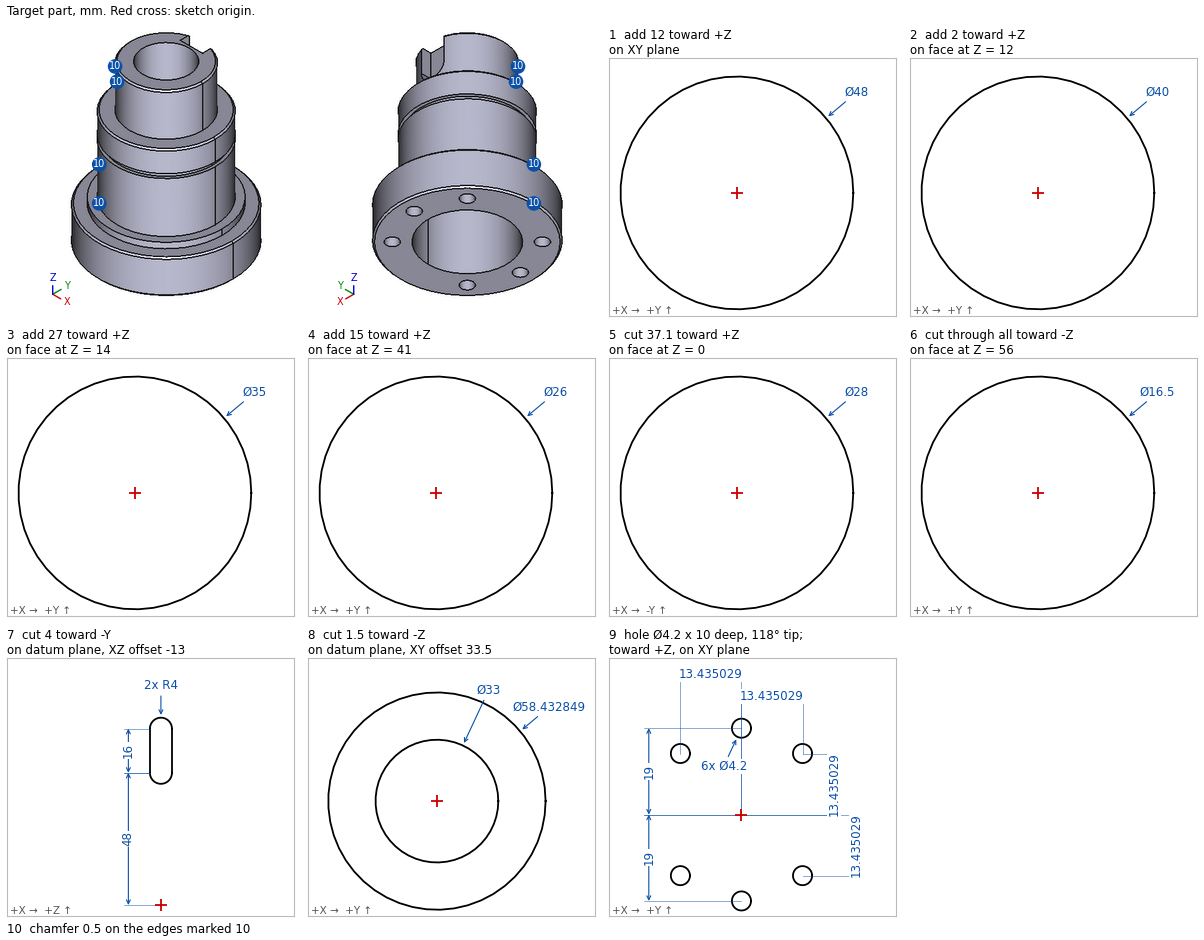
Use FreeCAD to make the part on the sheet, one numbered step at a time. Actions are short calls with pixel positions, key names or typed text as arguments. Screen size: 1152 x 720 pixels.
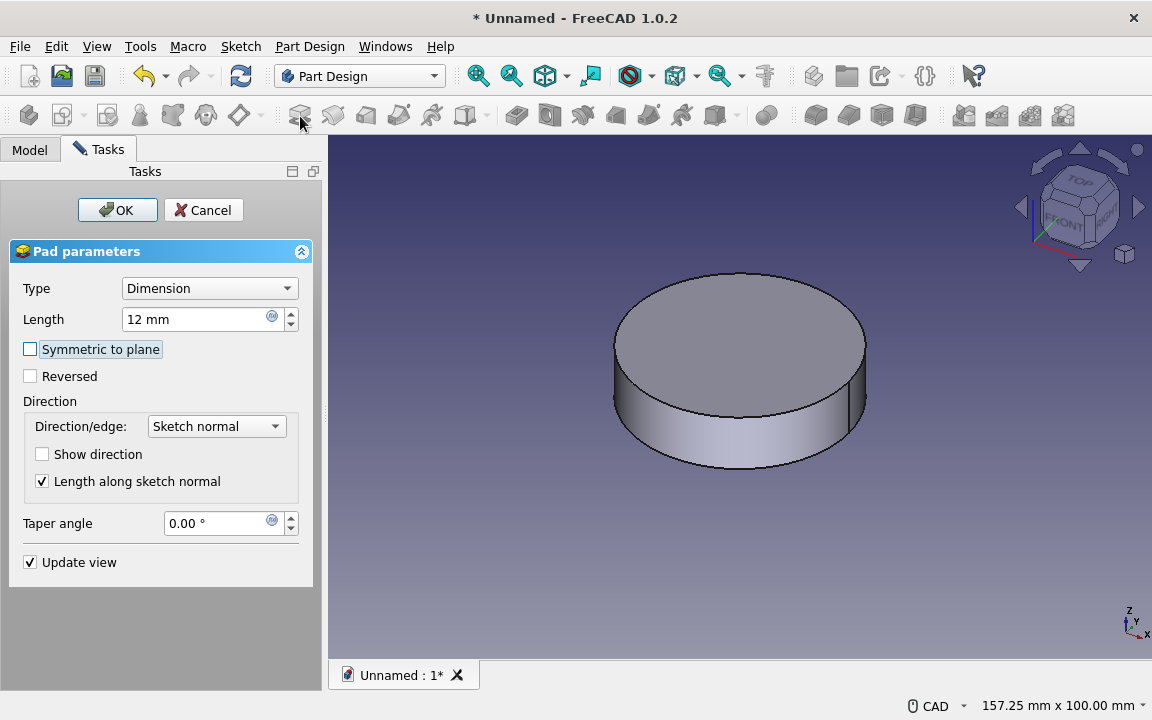
click(118, 210)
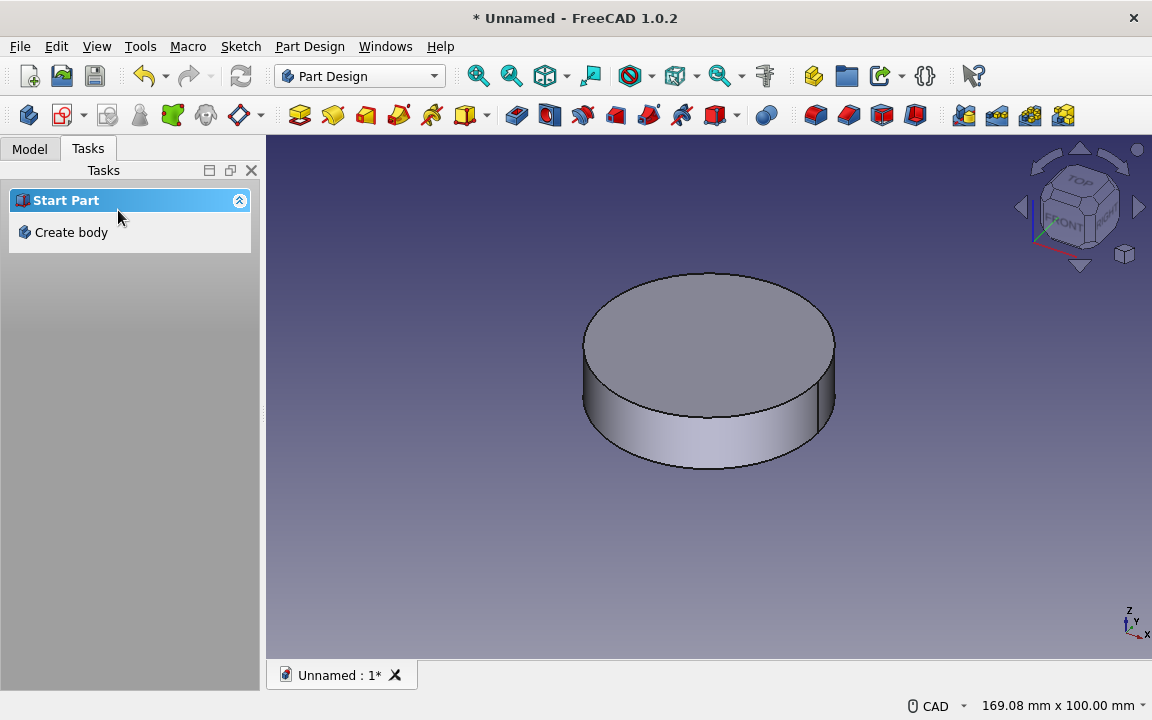
click(709, 344)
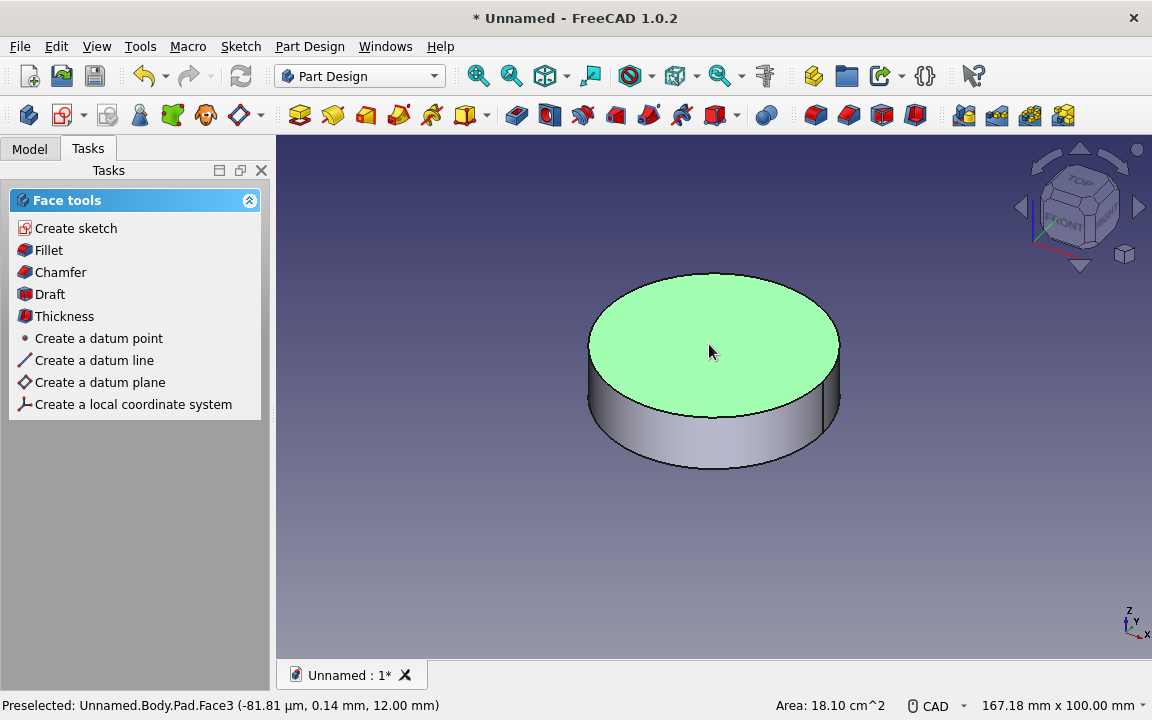
click(62, 116)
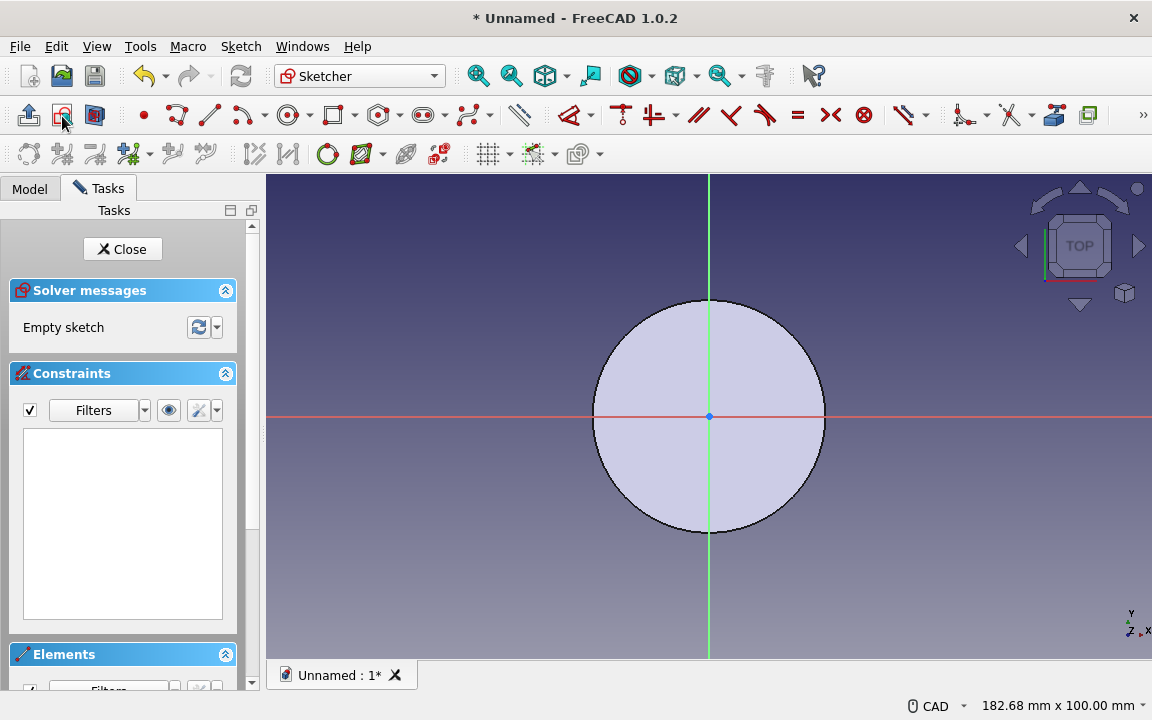
scroll(848, 416, up, 2)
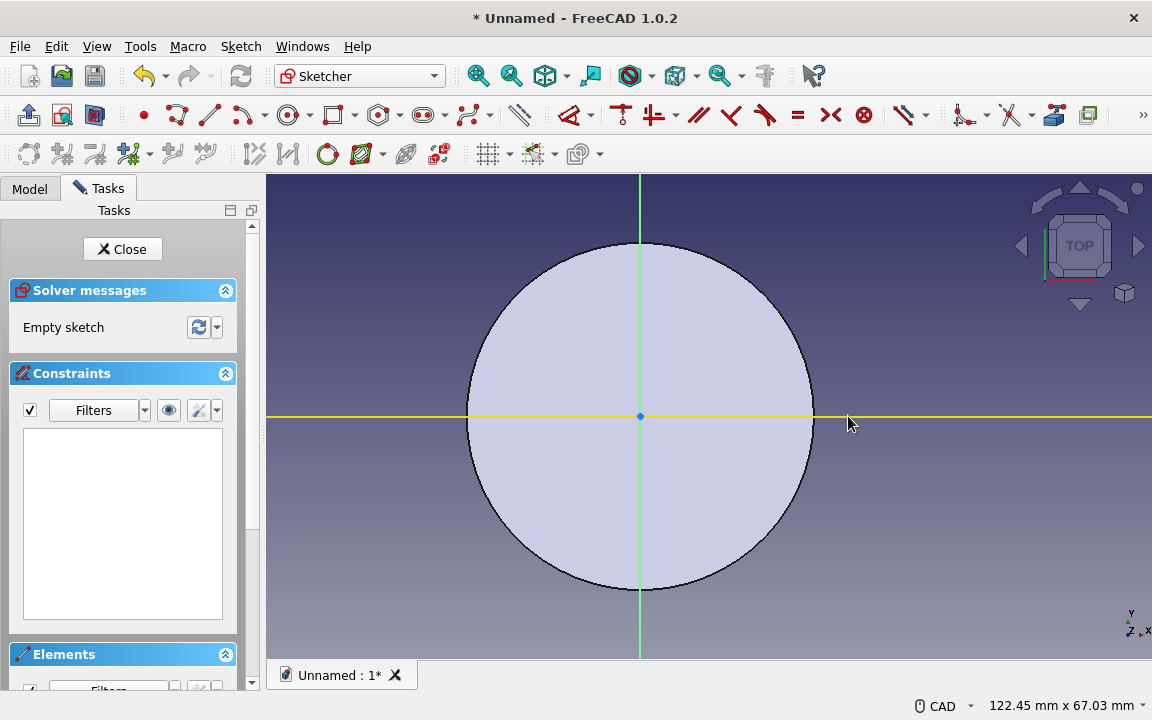
click(288, 116)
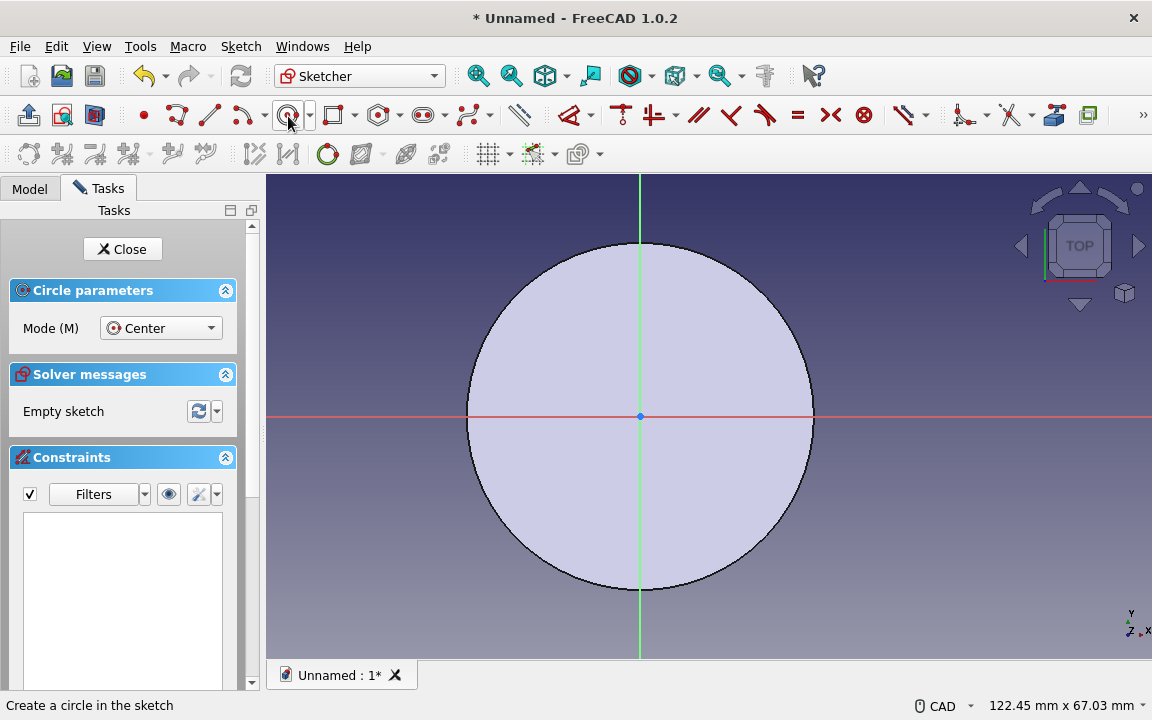
click(640, 416)
click(743, 314)
key(Escape)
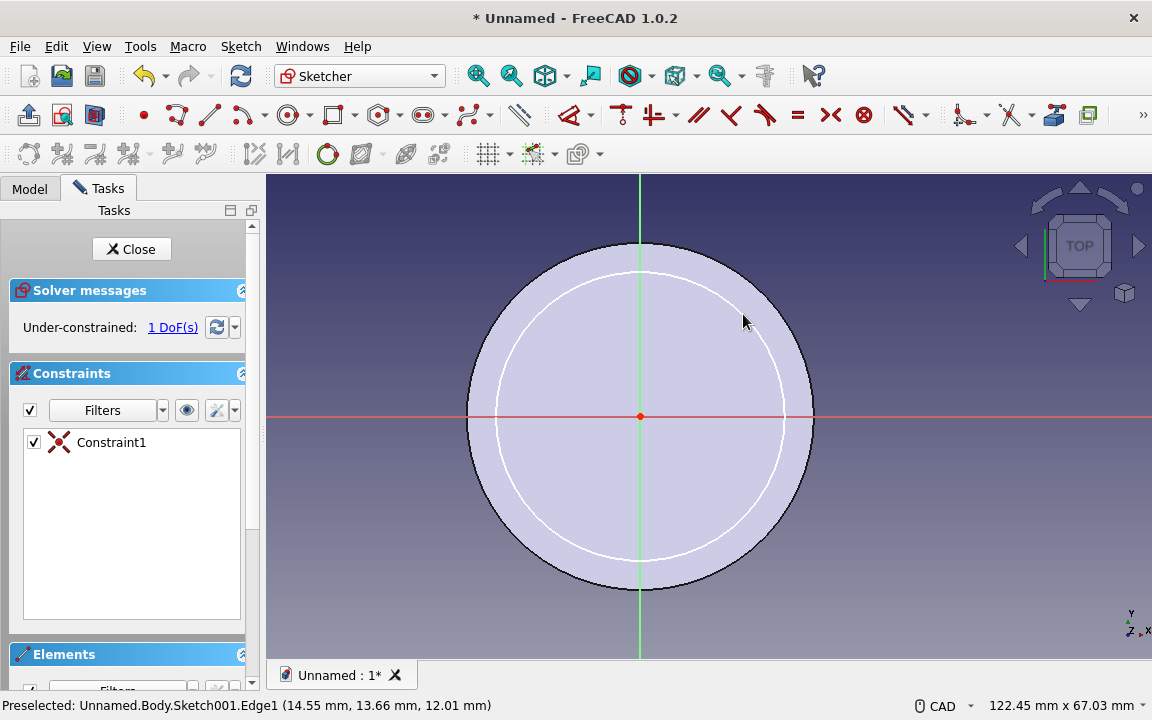
click(742, 314)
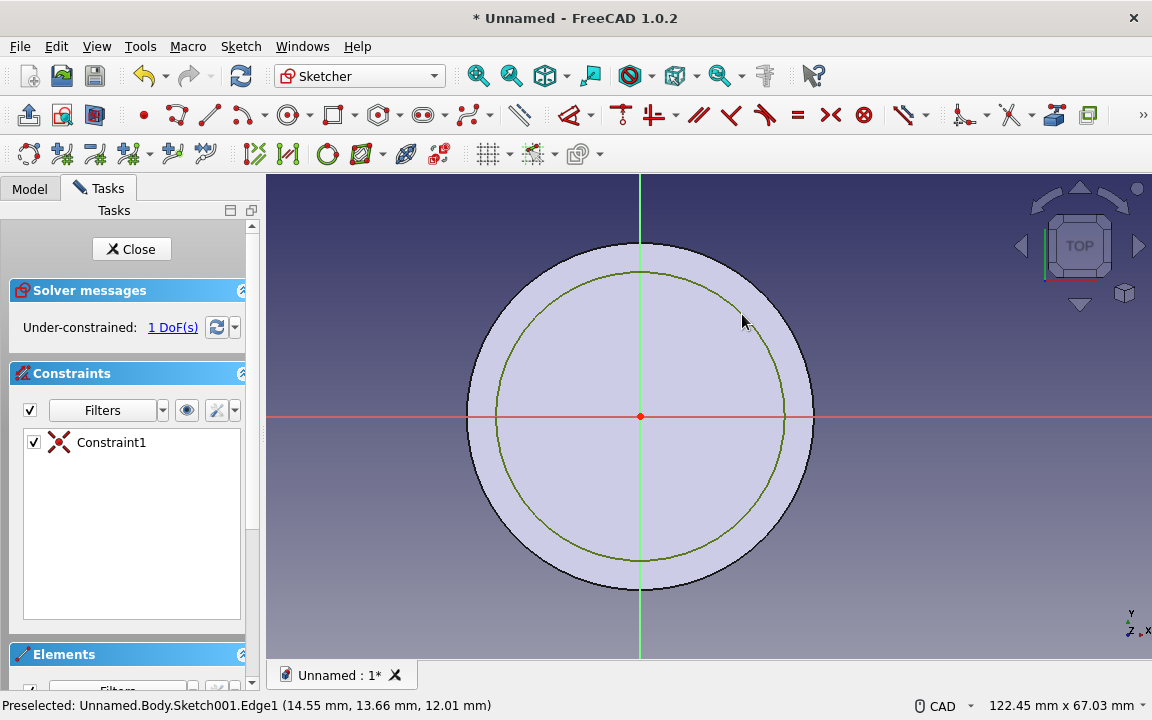
key(k)
key(o)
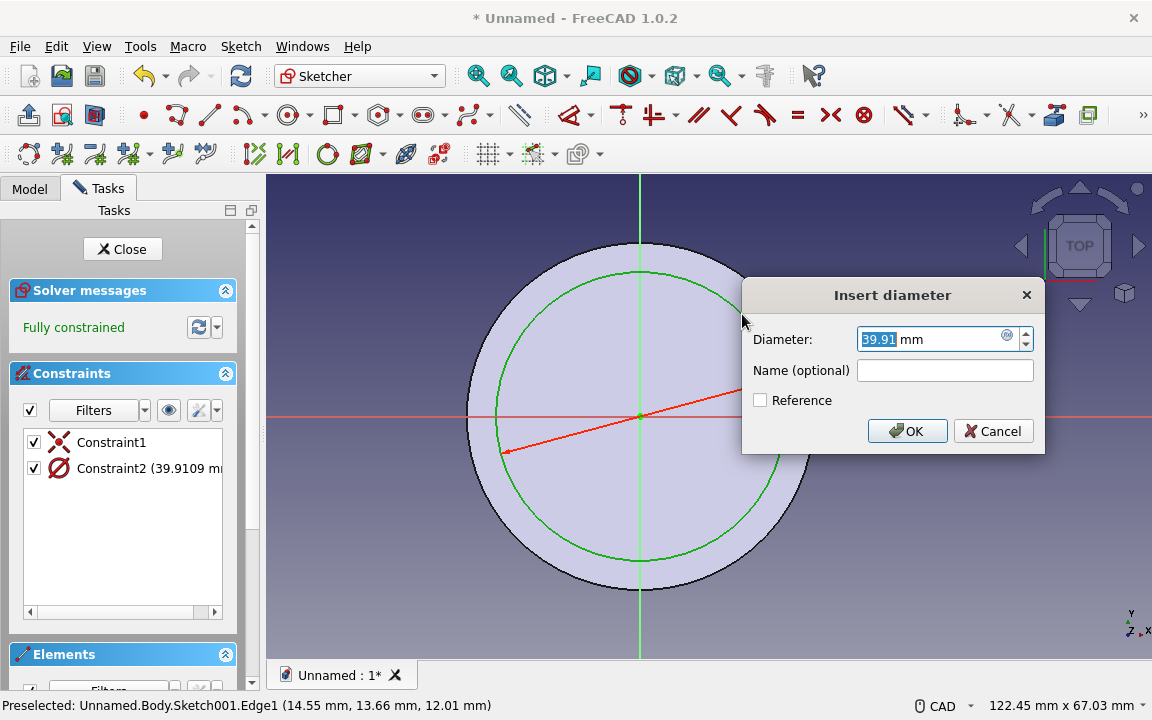
text(40)
key(Return)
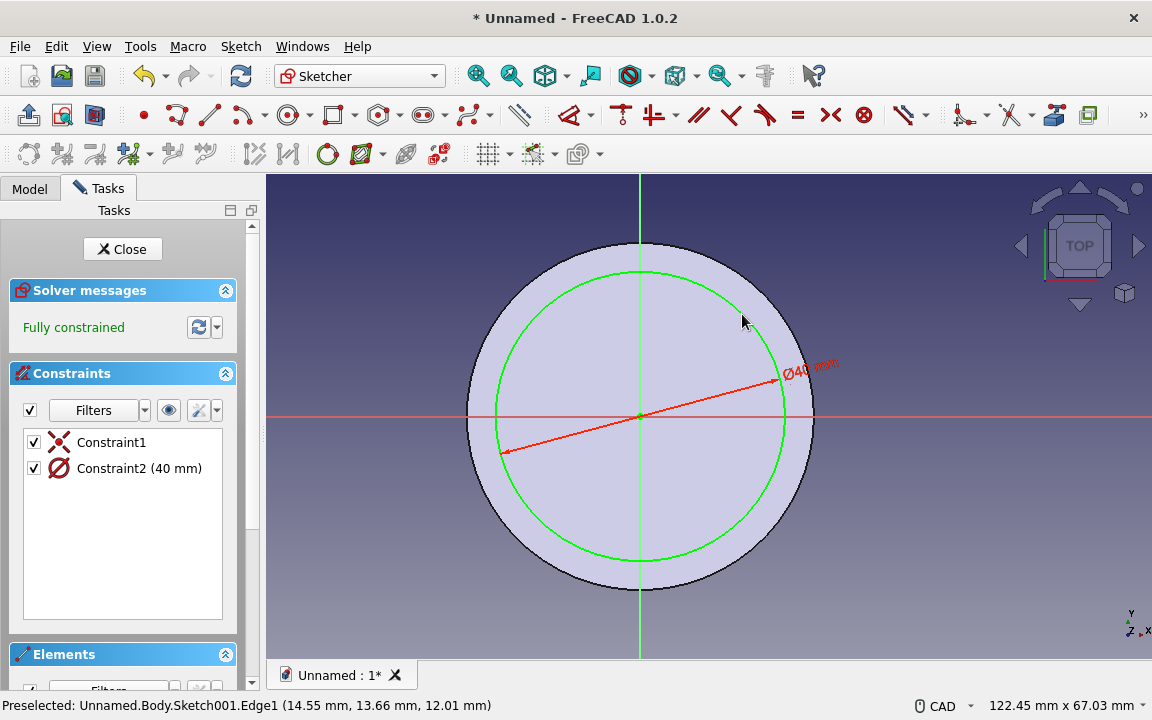
click(123, 249)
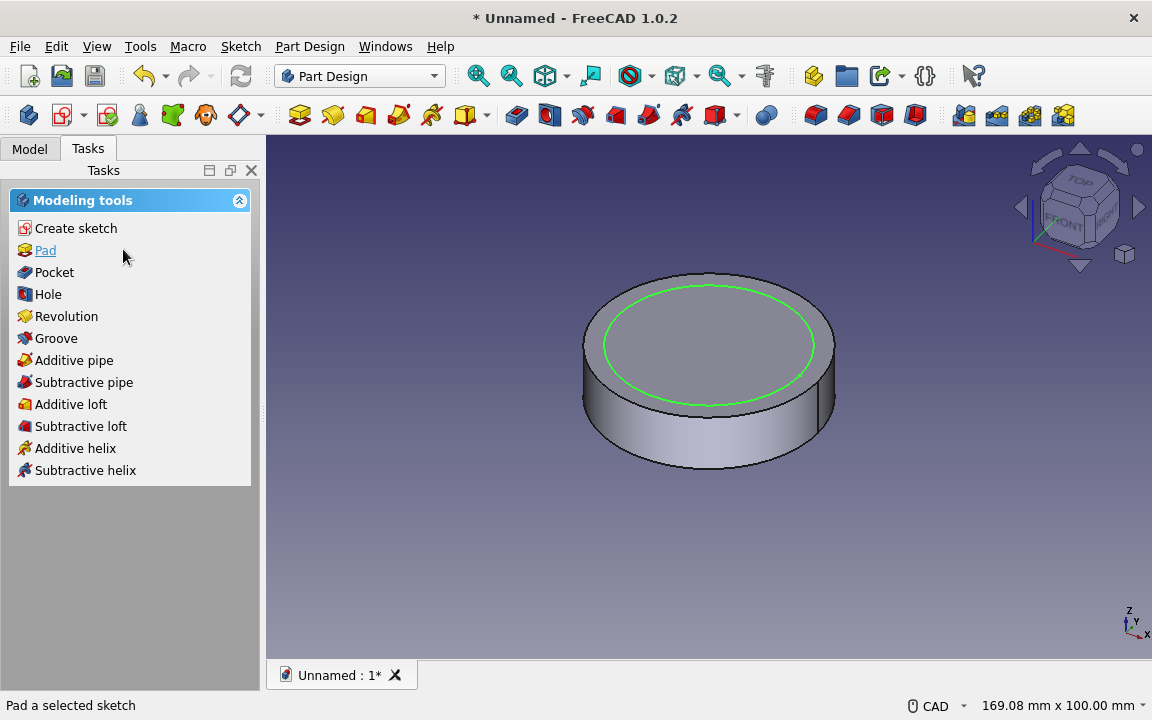
click(300, 116)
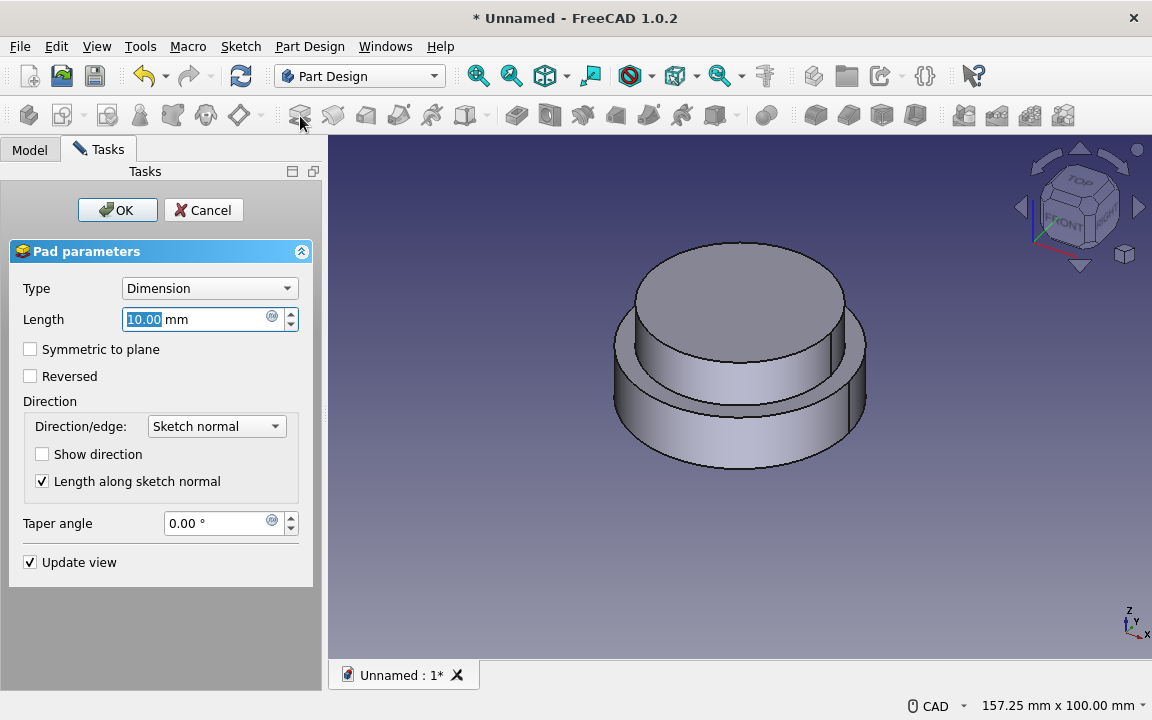
text(2)
key(Tab)